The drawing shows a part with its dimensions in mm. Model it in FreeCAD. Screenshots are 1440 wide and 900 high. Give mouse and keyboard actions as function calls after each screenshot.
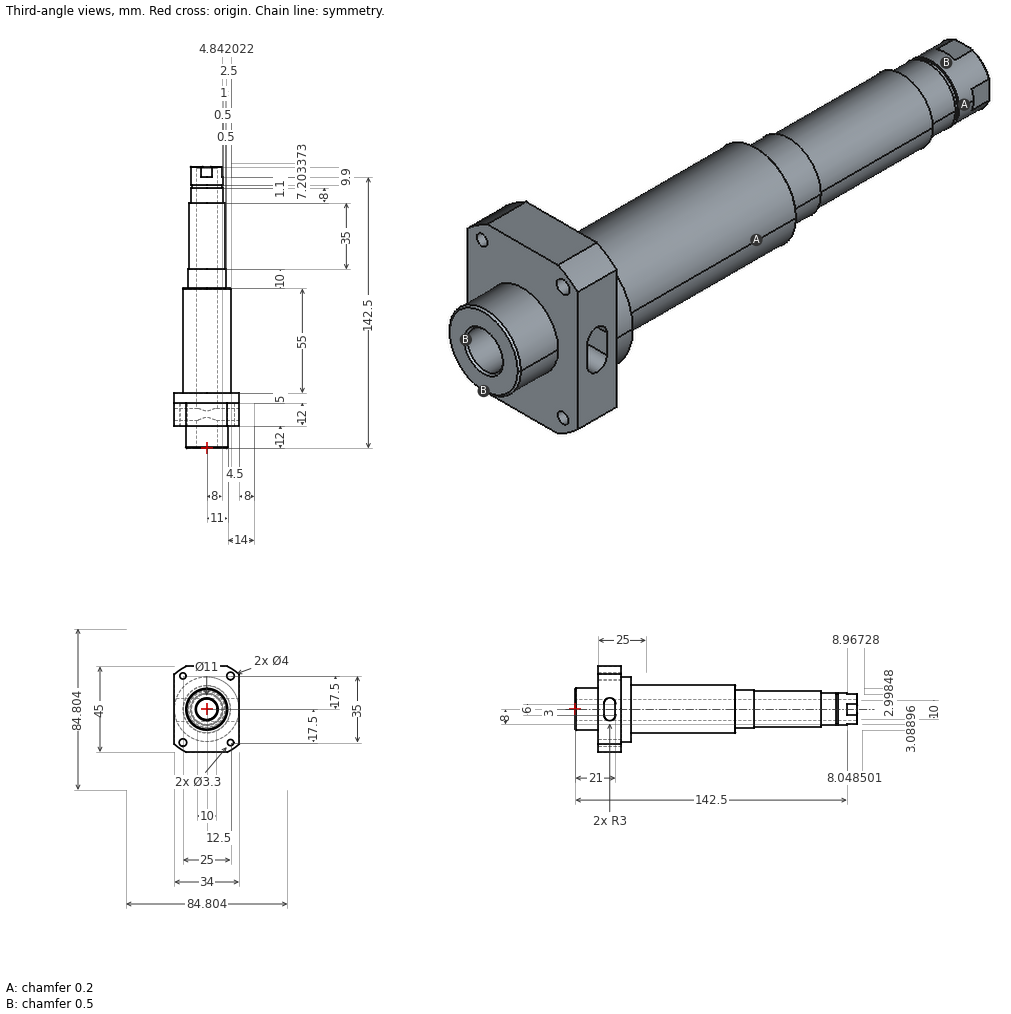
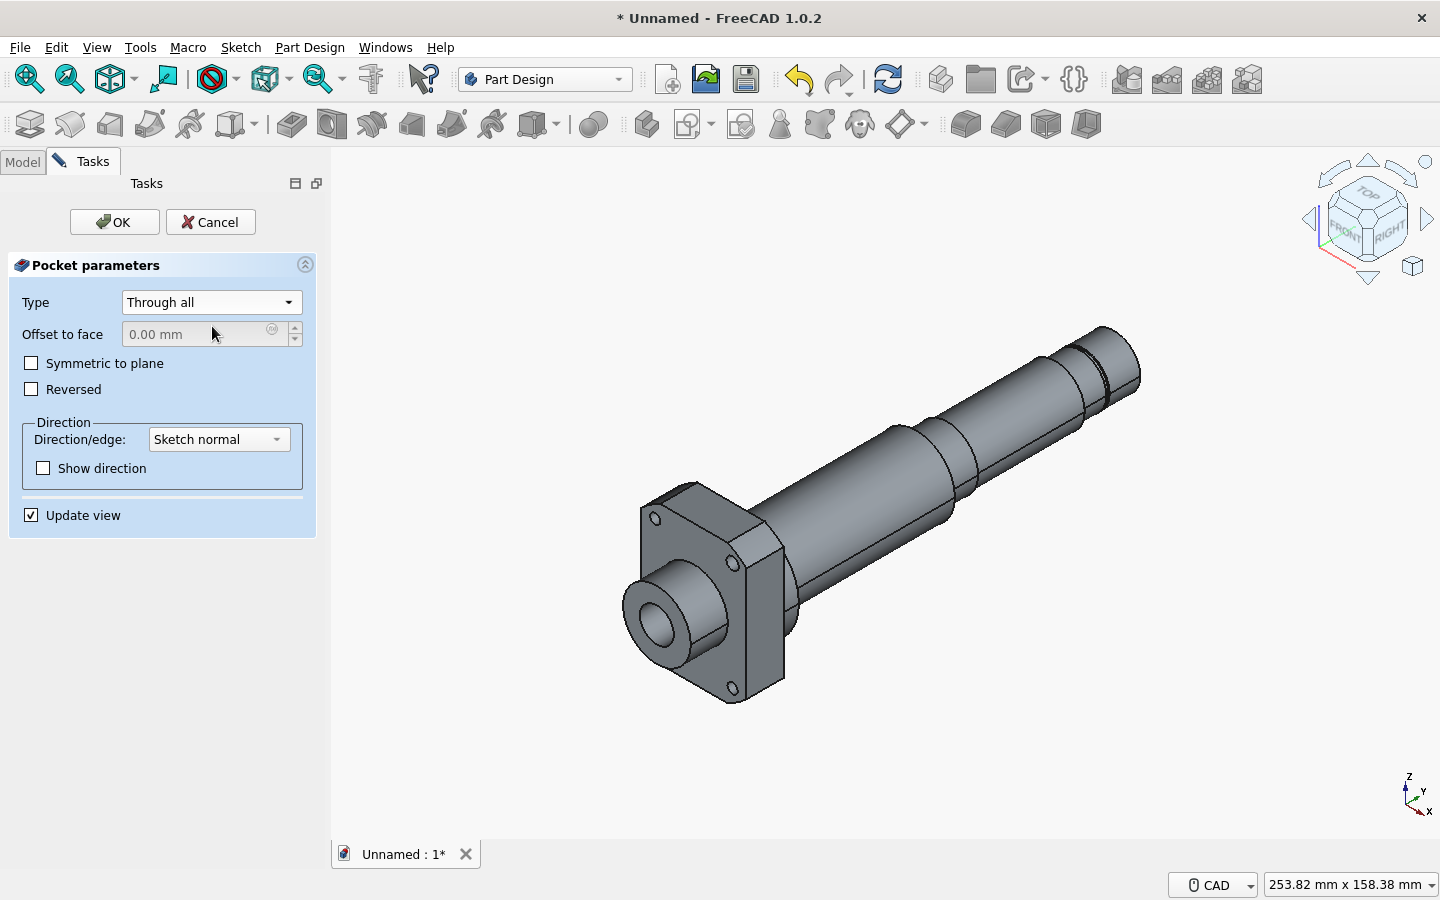
click(115, 222)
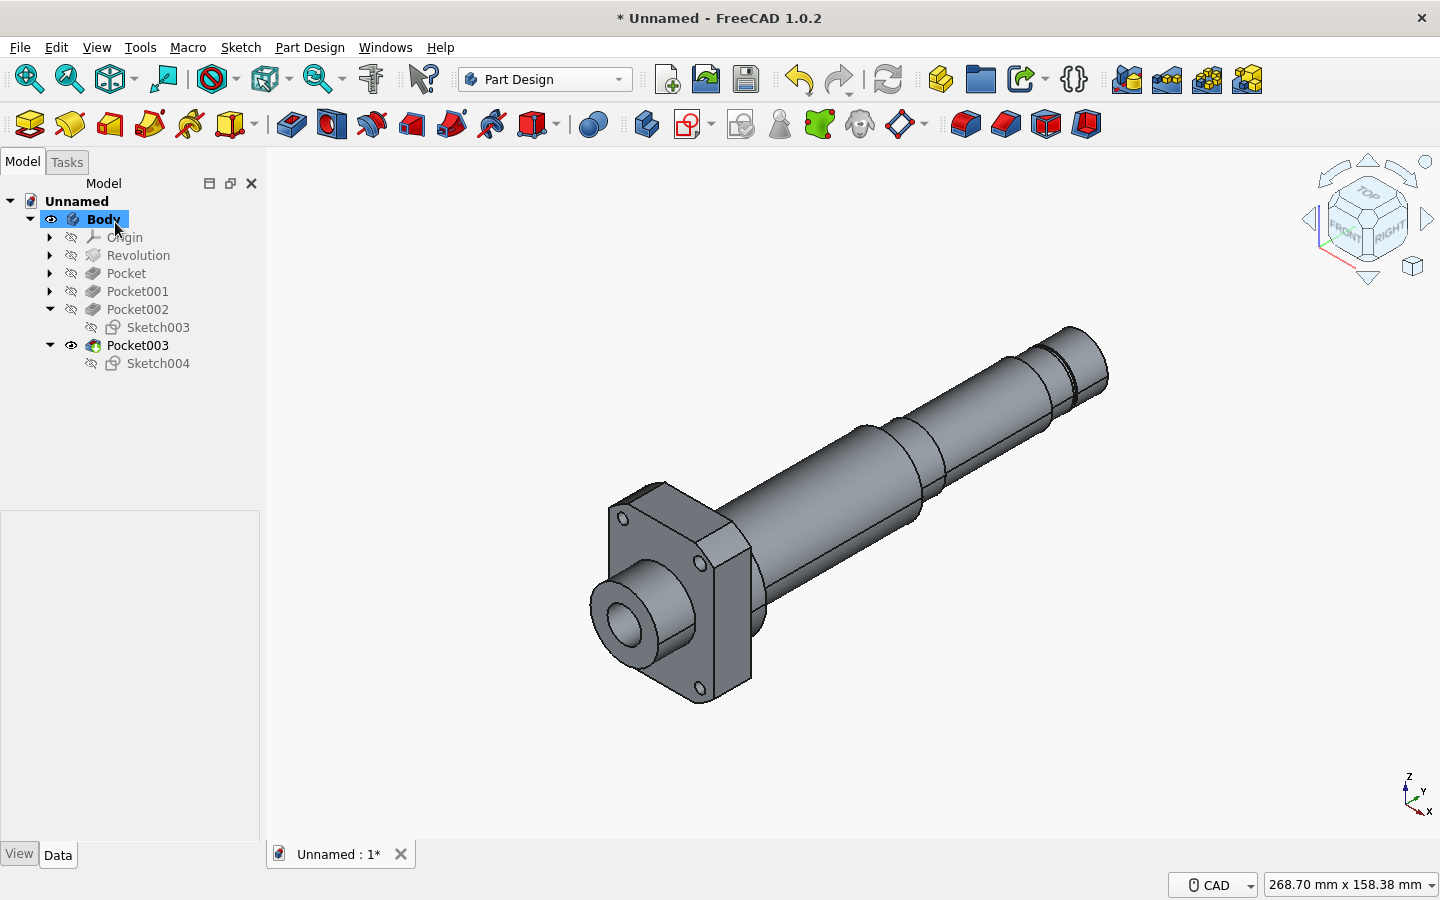
key(2)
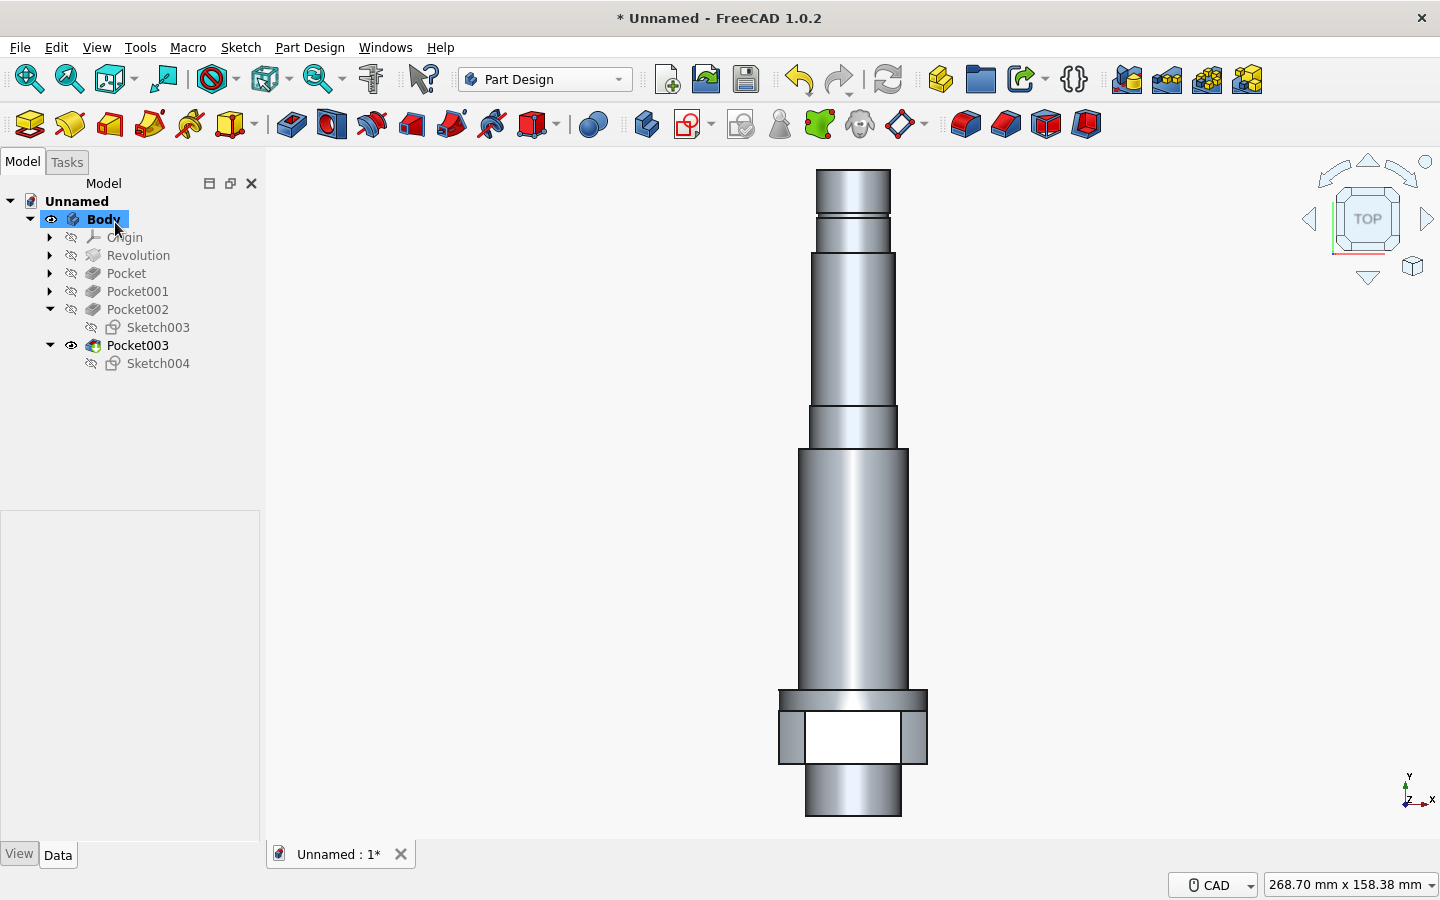
click(809, 448)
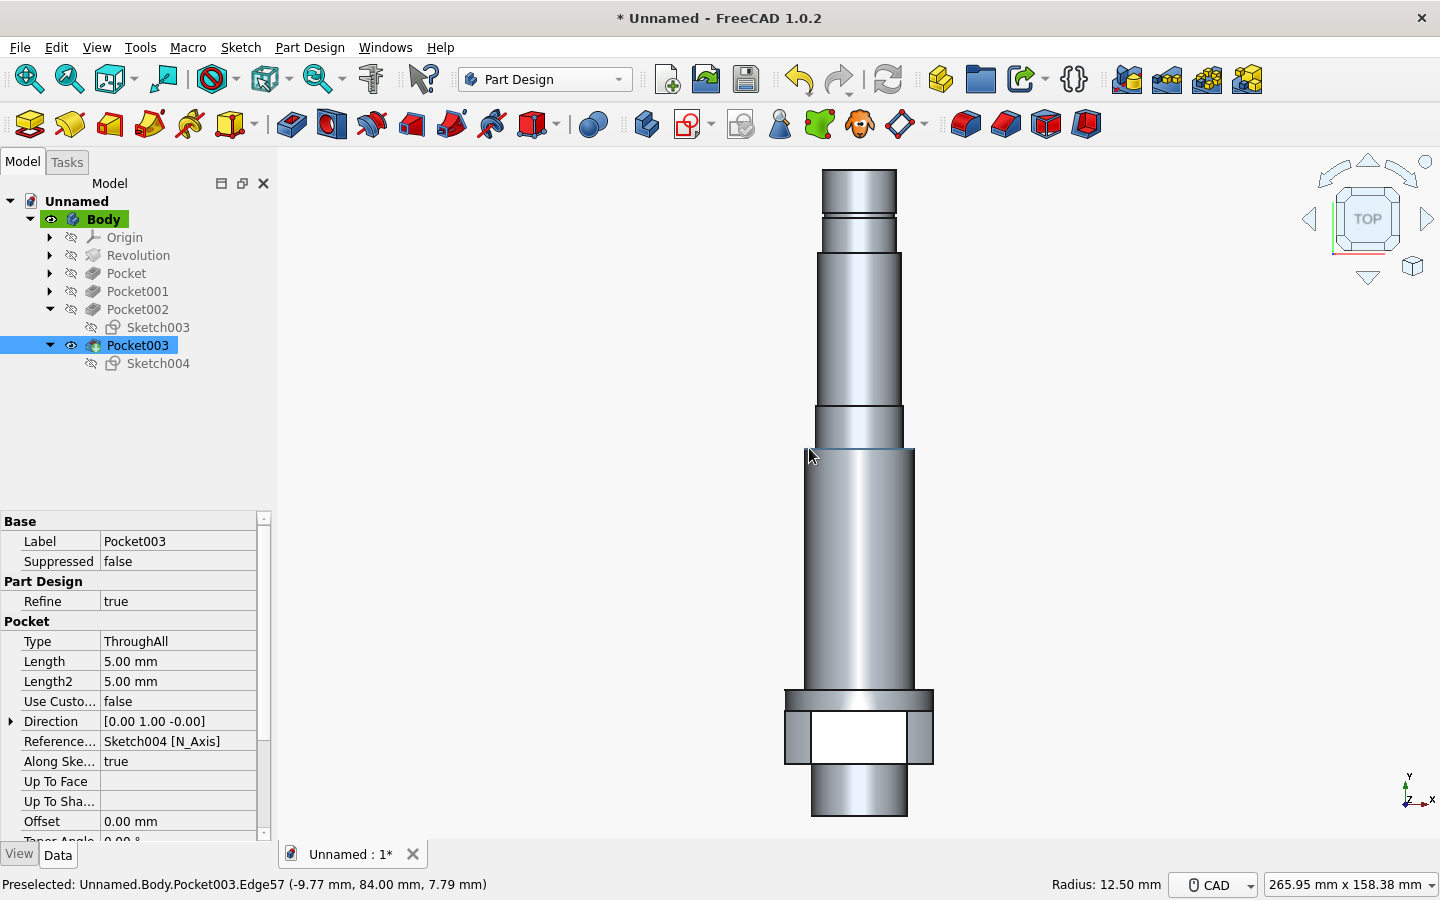
key(0)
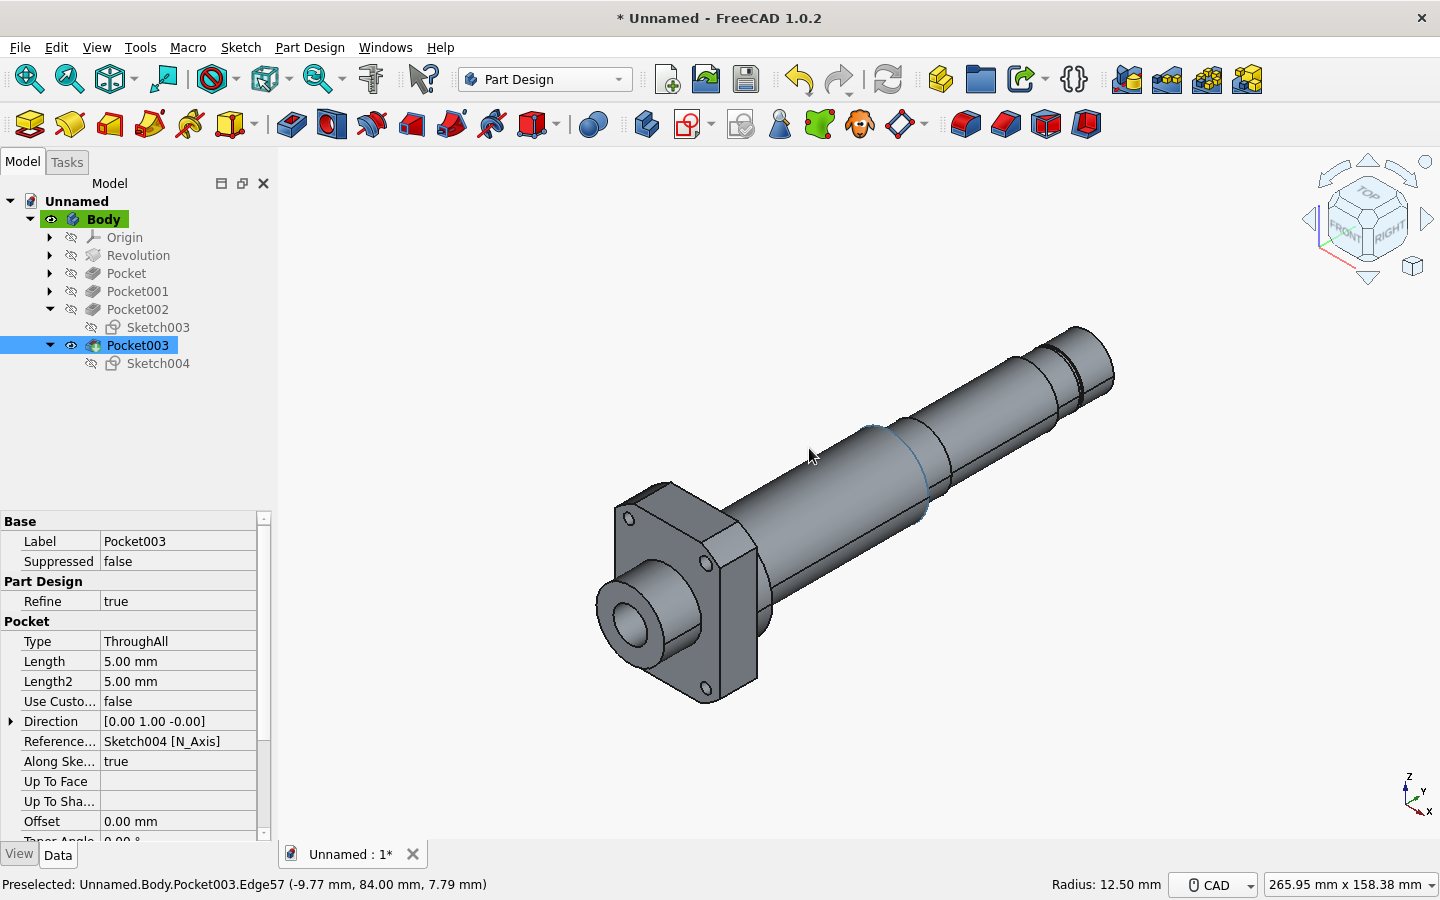
key(1)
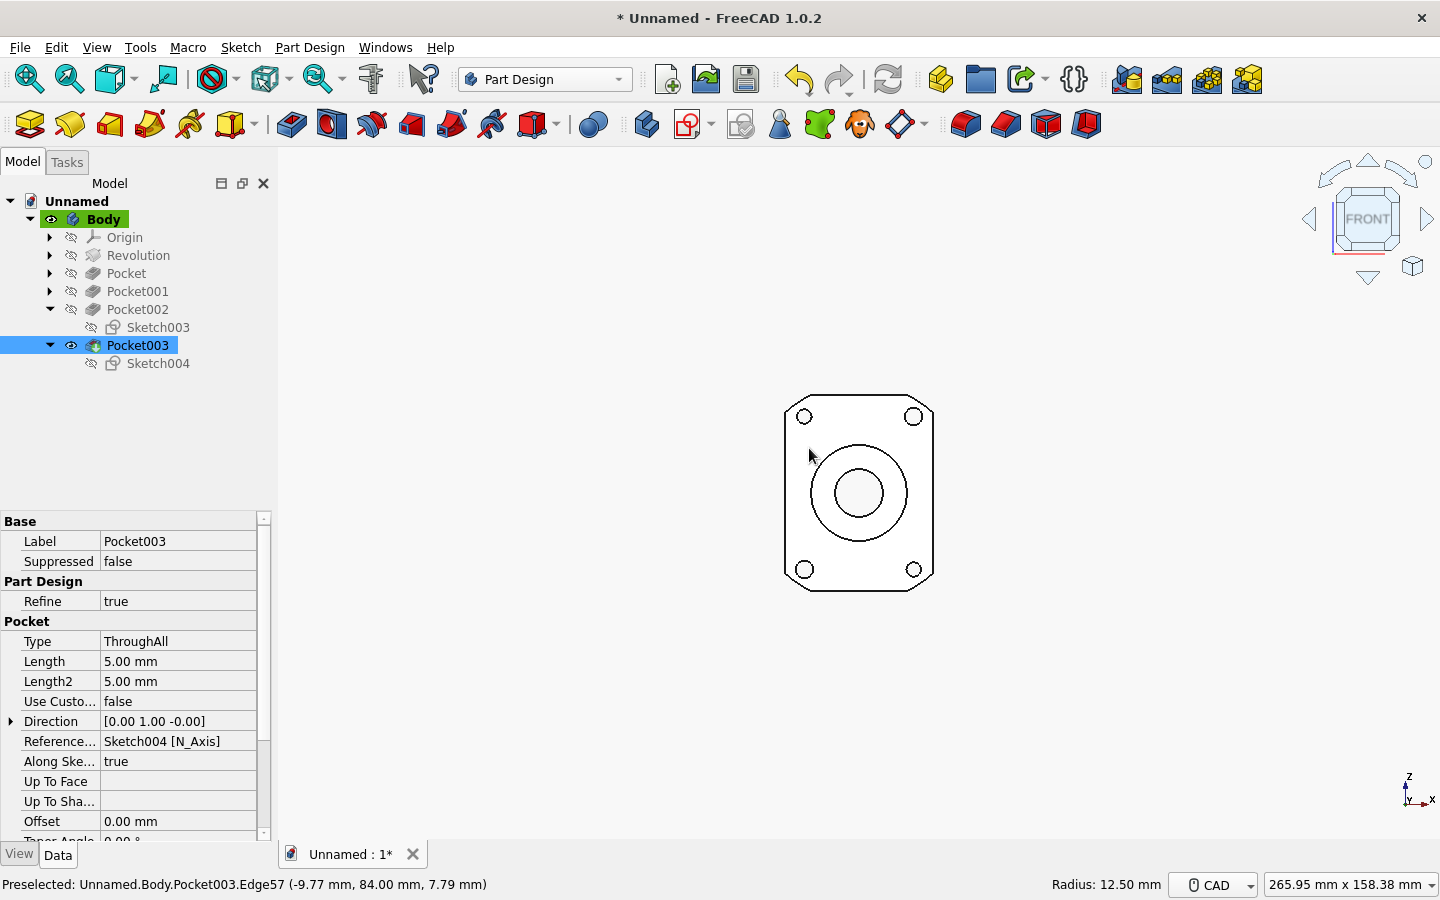
key(v)
key(f)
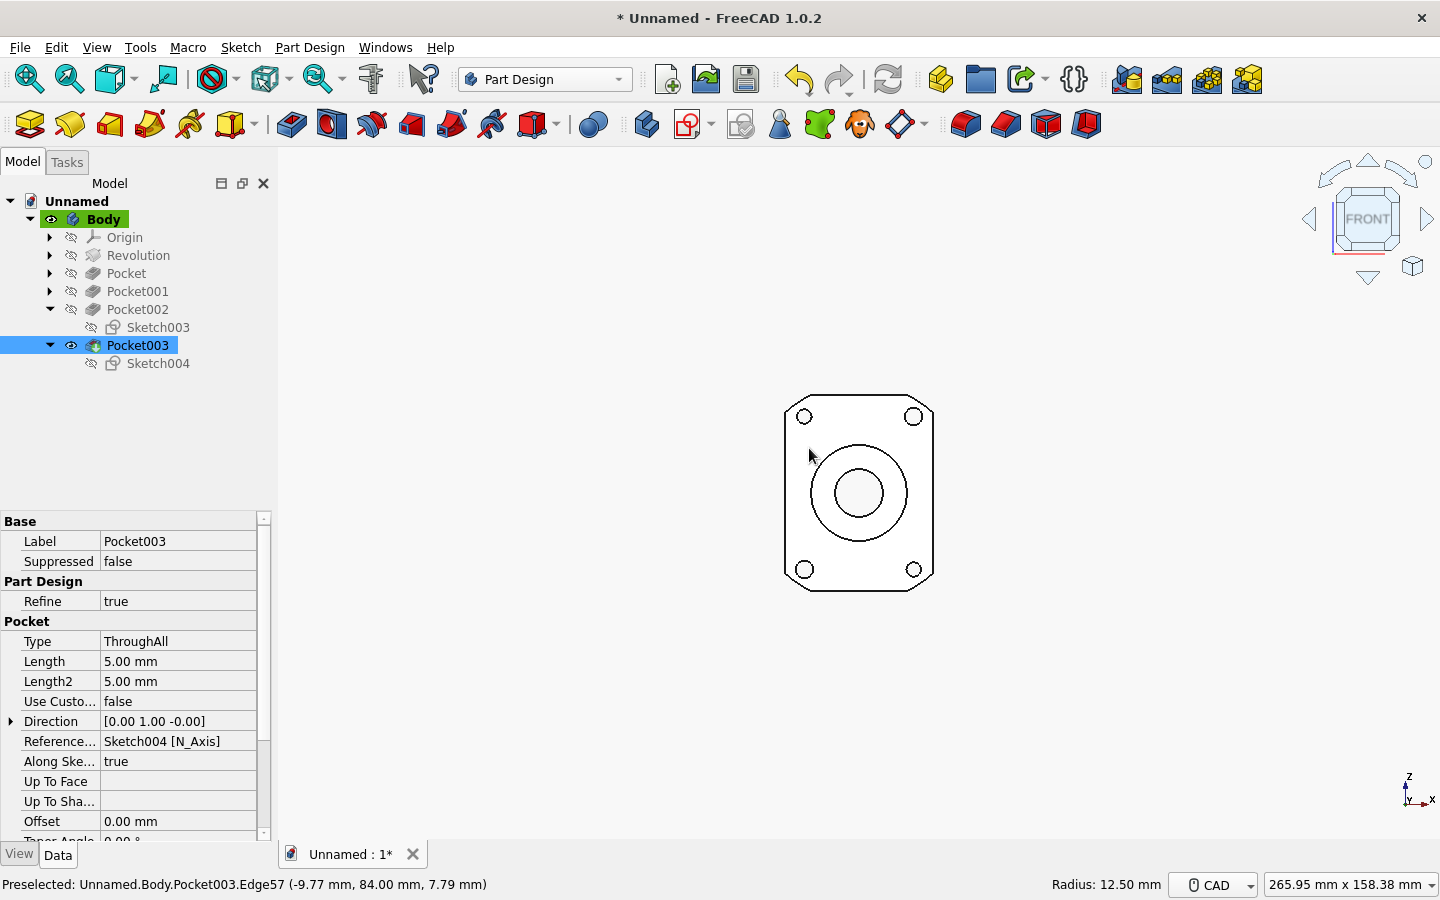
key(3)